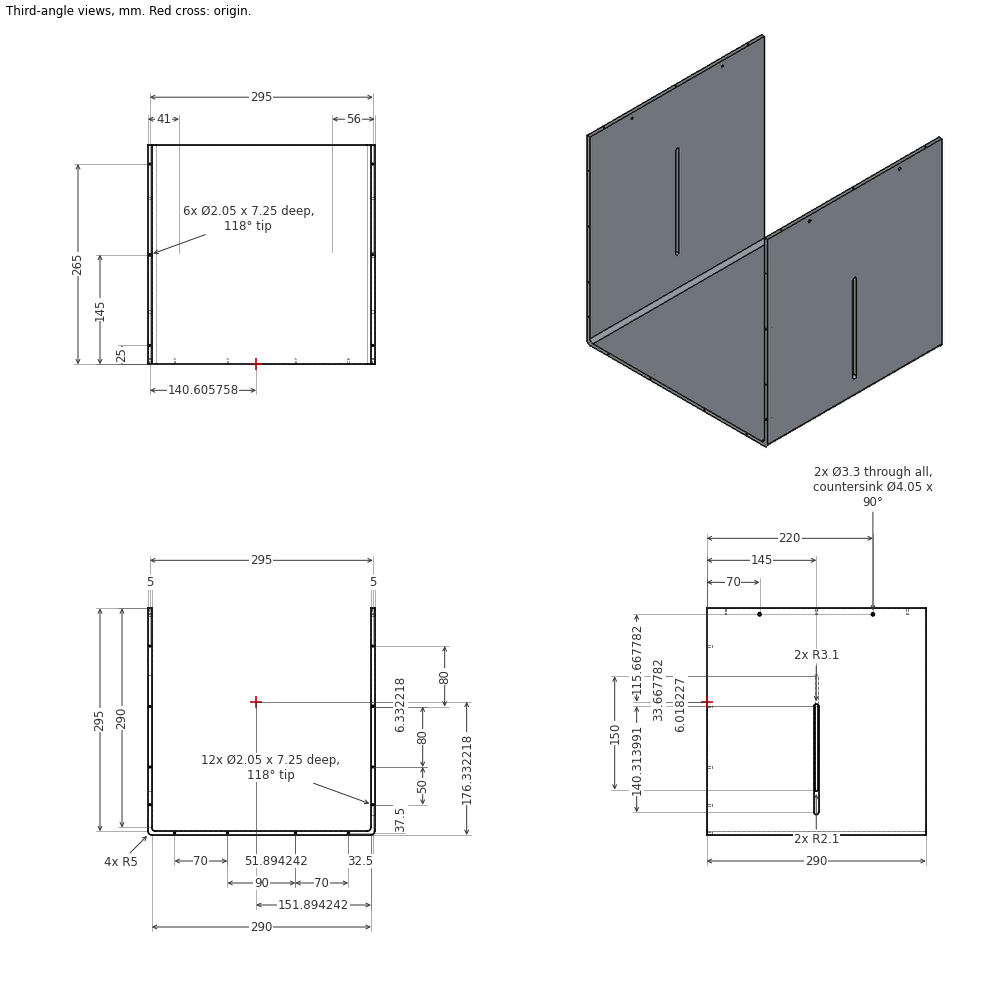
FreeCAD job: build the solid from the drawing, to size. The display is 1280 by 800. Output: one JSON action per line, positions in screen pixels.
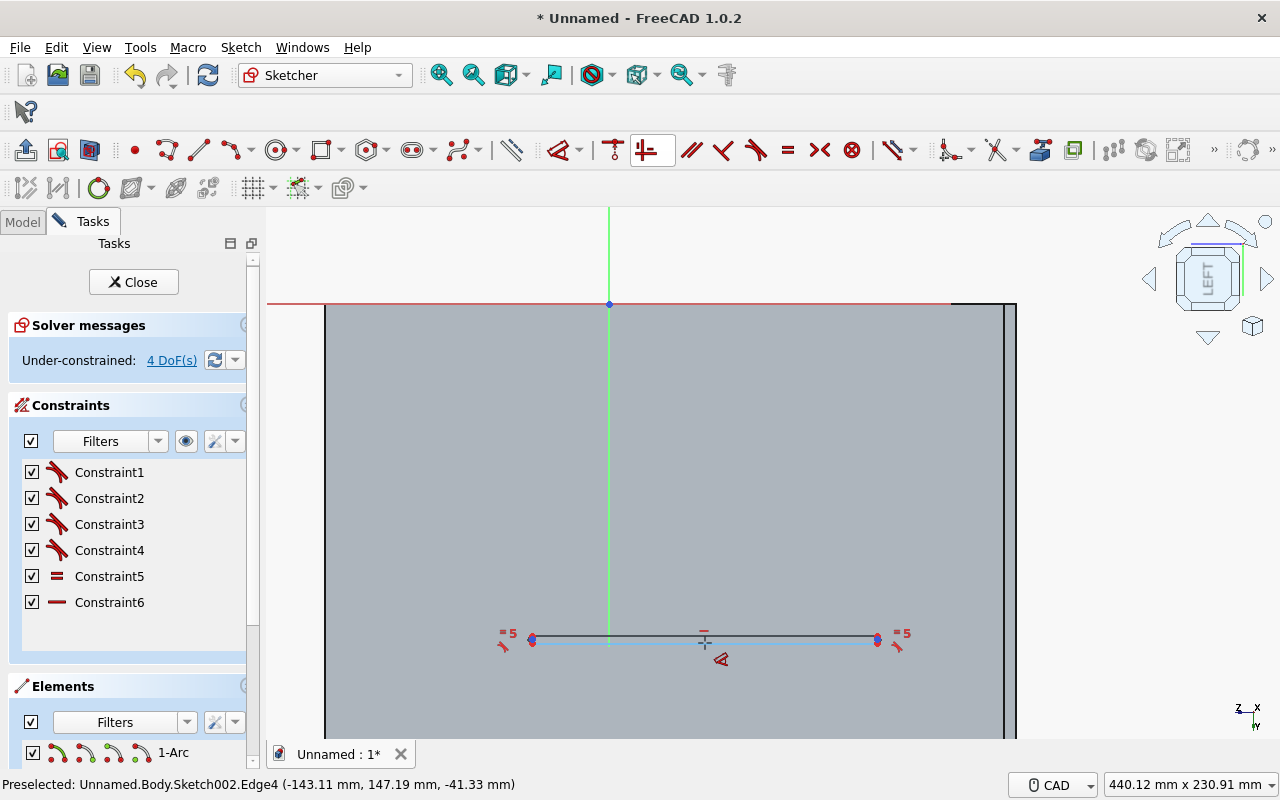
{"action": "scroll", "coordinate": [529, 638], "scroll_direction": "up", "scroll_amount": 11}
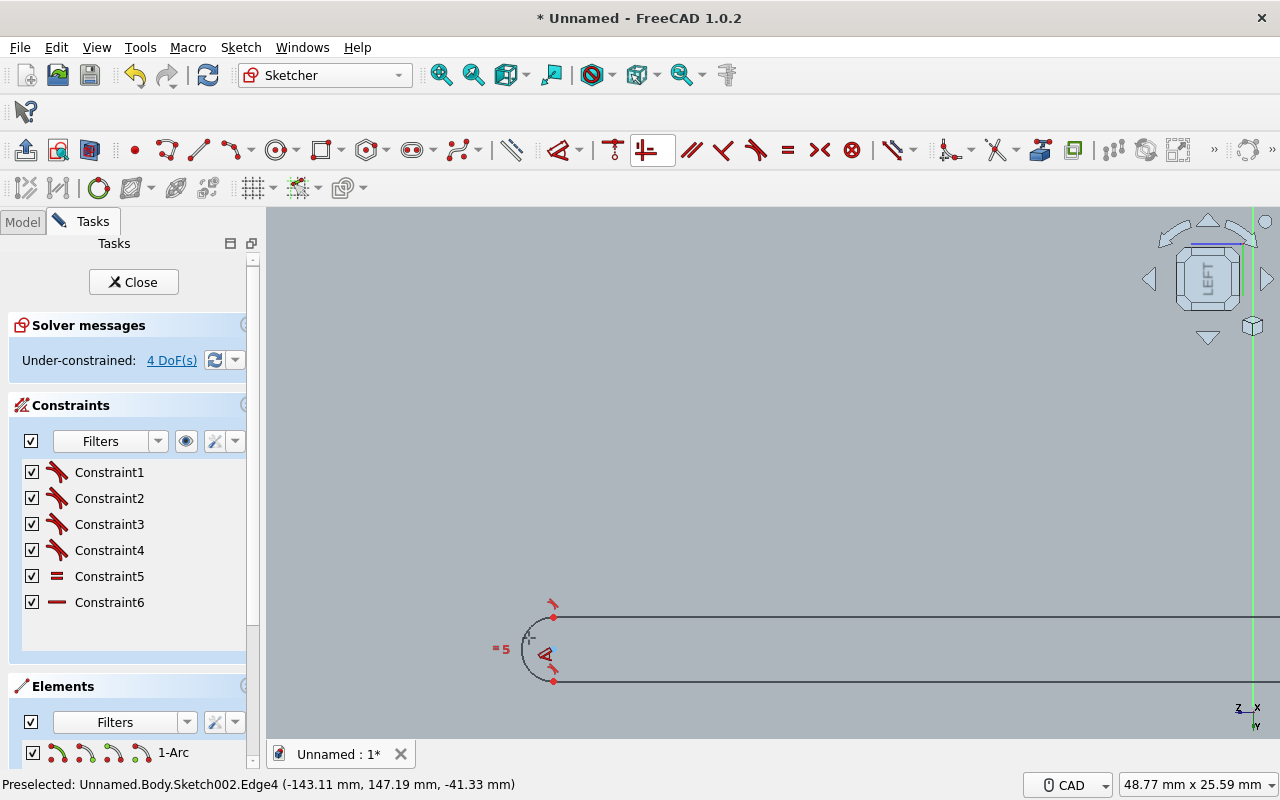
{"action": "left_click", "coordinate": [528, 631]}
{"action": "left_click", "coordinate": [502, 612]}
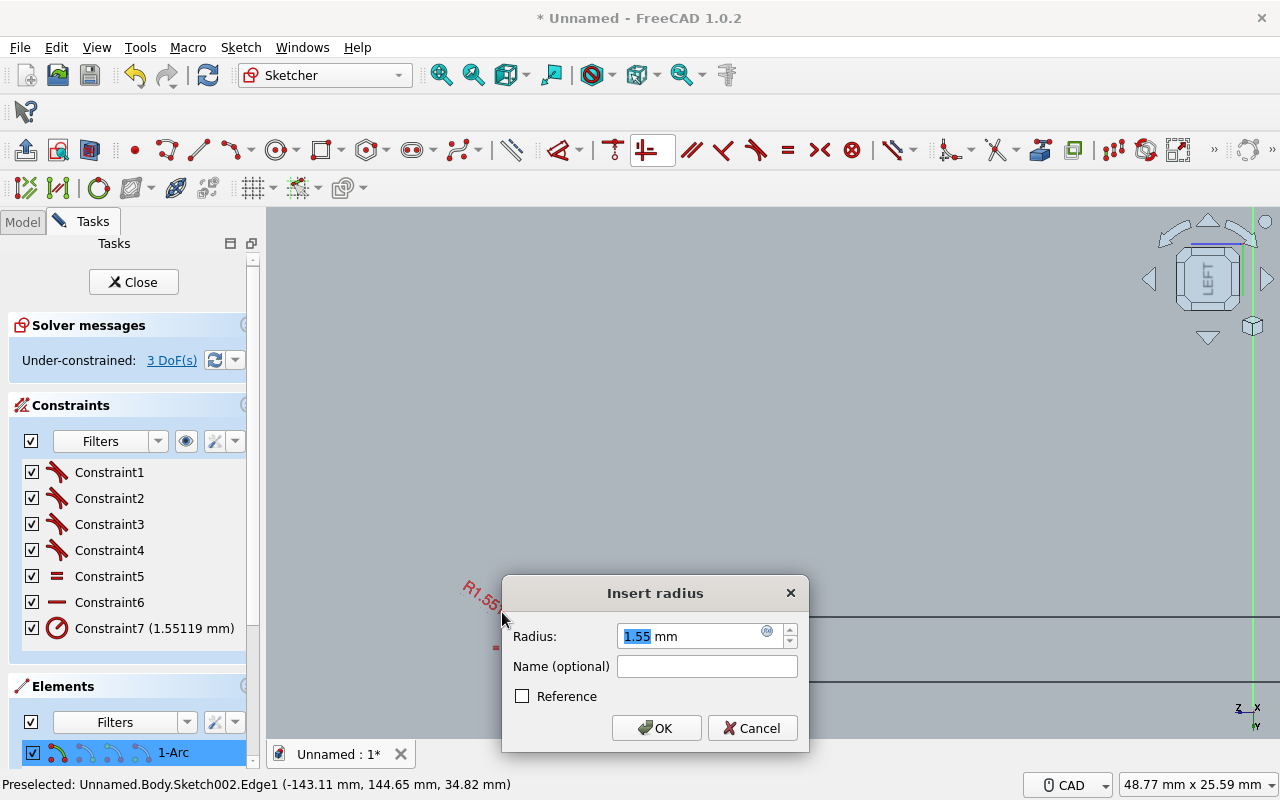
{"action": "type", "text": "2.1"}
{"action": "key", "text": "Return"}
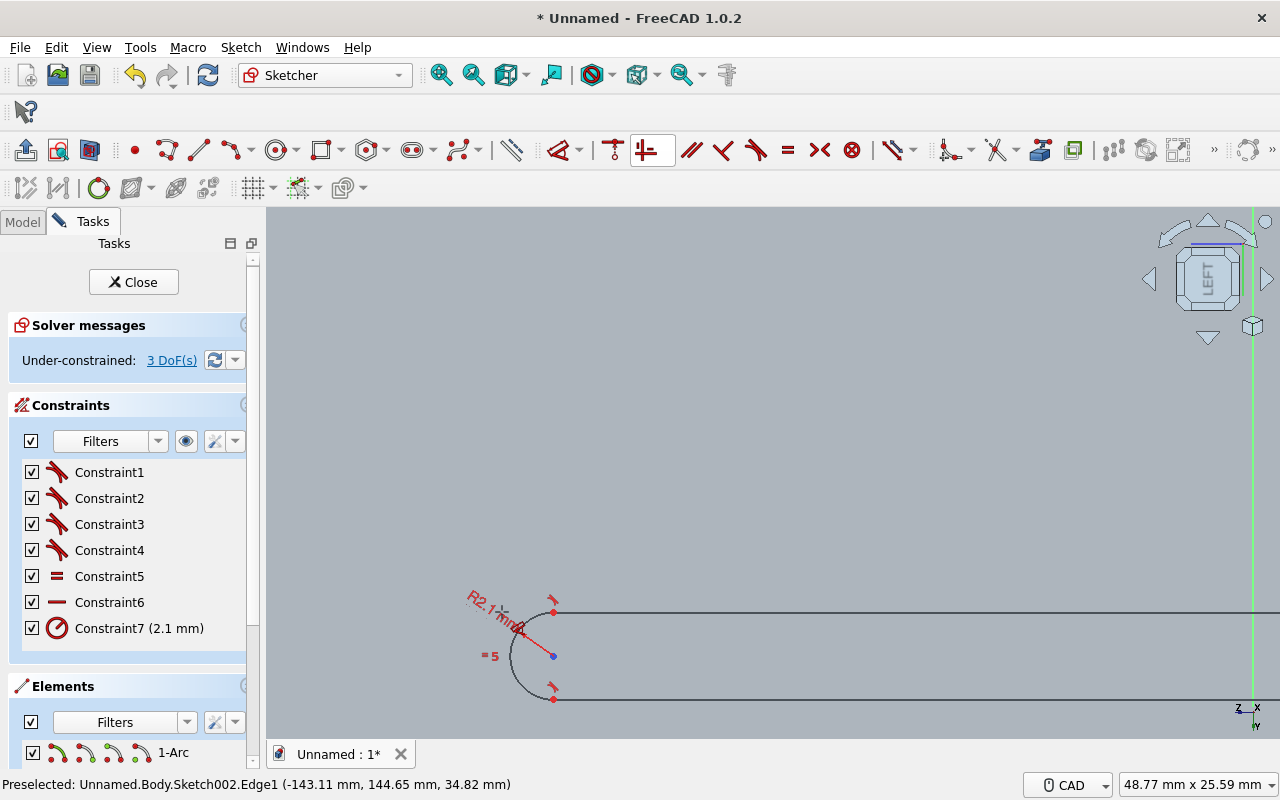
{"action": "scroll", "coordinate": [529, 638], "scroll_direction": "down", "scroll_amount": 11}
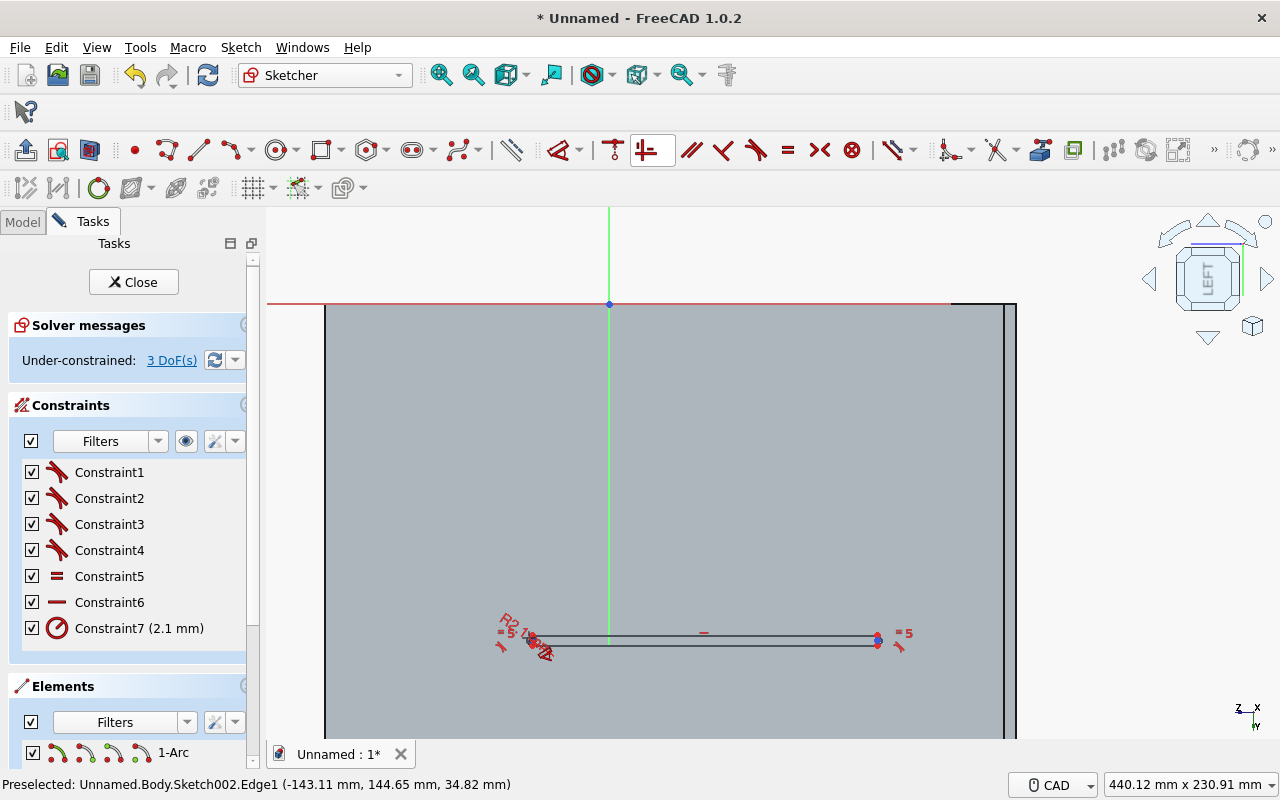
{"action": "scroll", "coordinate": [635, 636], "scroll_direction": "up", "scroll_amount": 2}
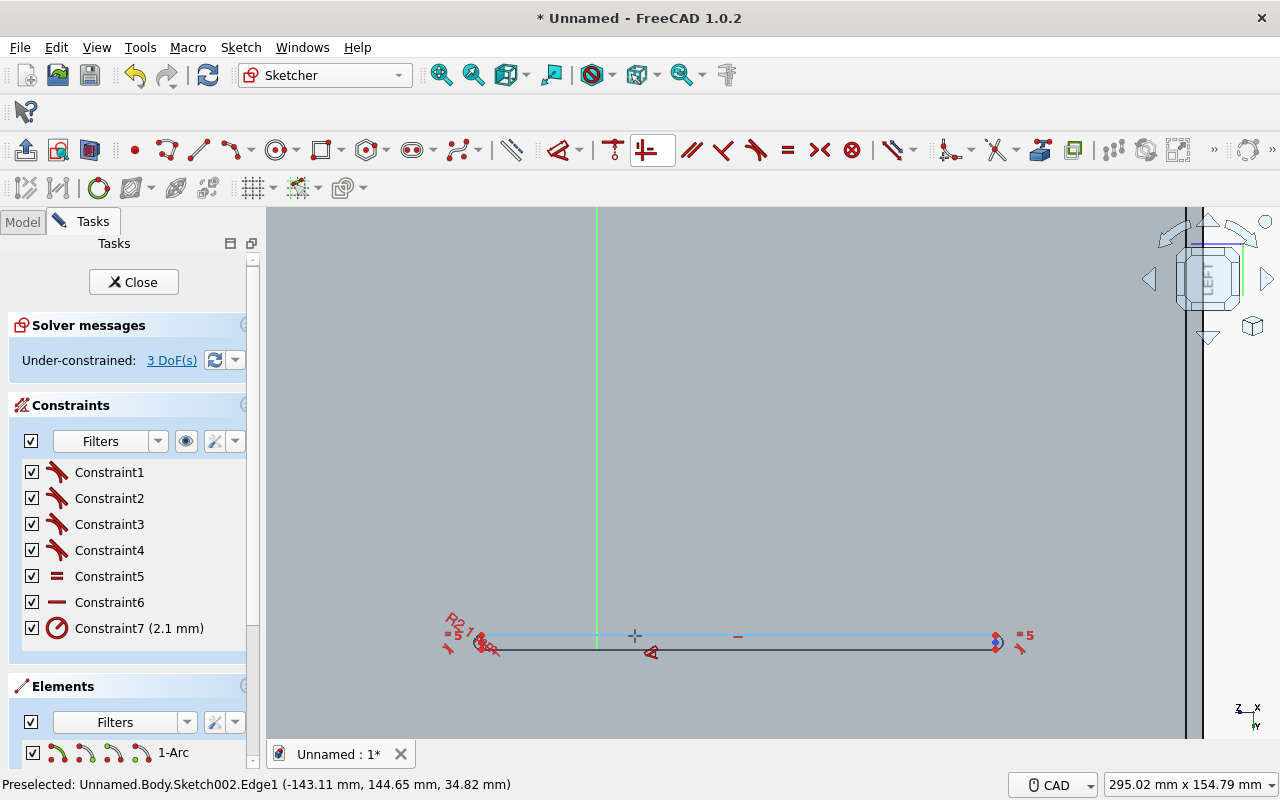
{"action": "left_click", "coordinate": [636, 635]}
{"action": "left_click", "coordinate": [739, 669]}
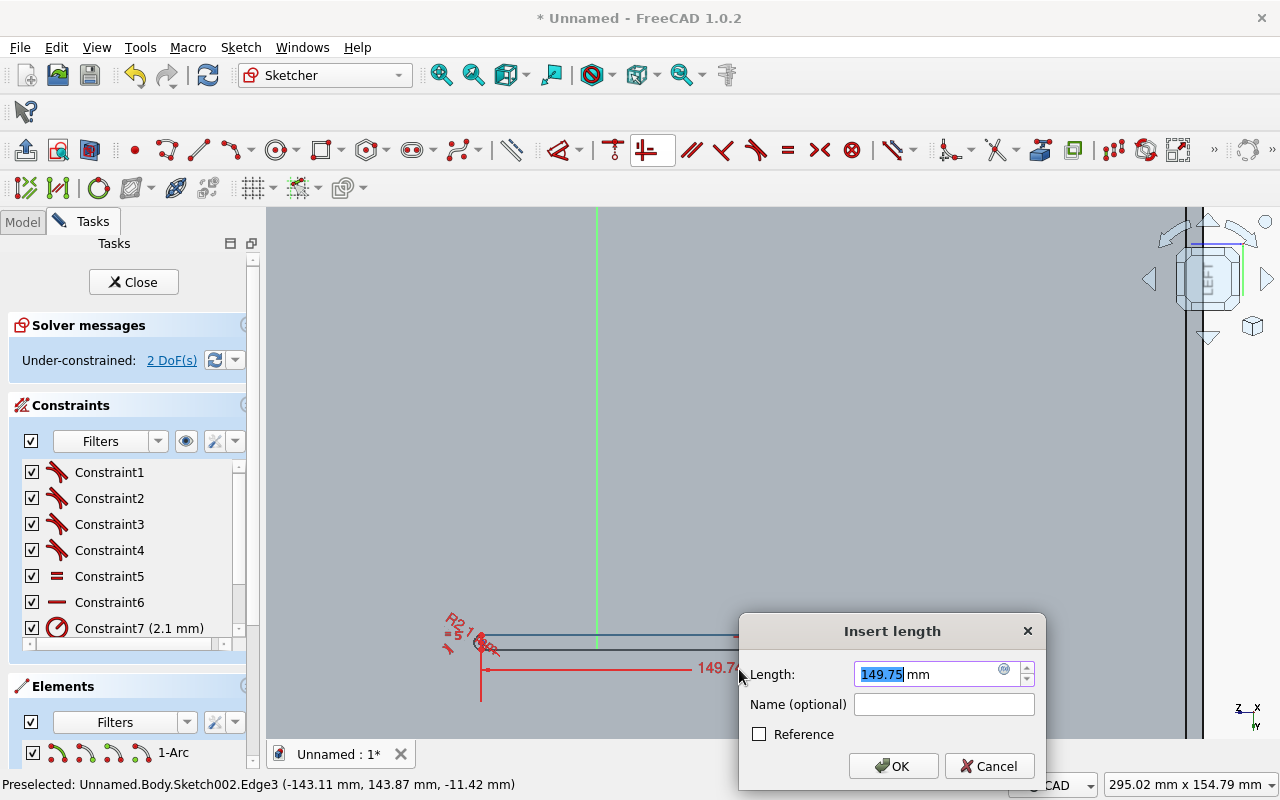
{"action": "type", "text": "150"}
{"action": "key", "text": "Return"}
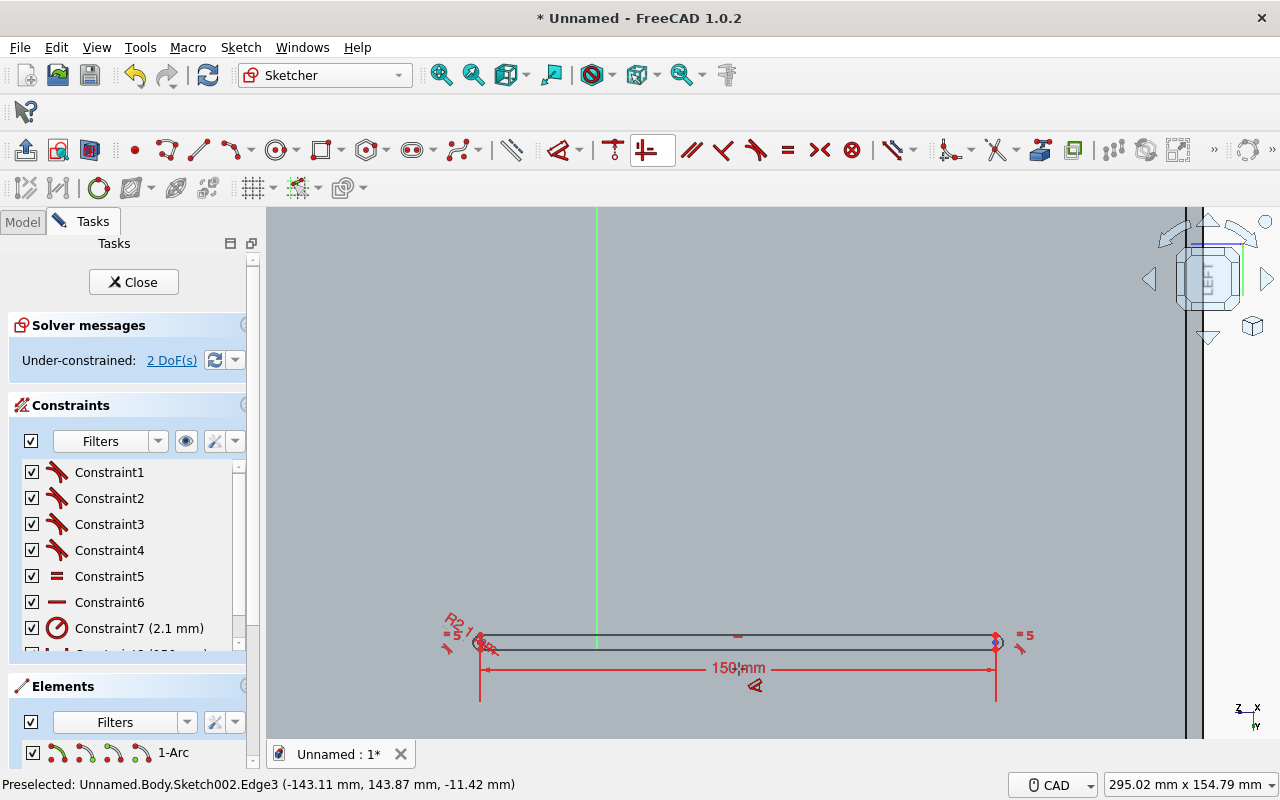
{"action": "scroll", "coordinate": [480, 643], "scroll_direction": "up", "scroll_amount": 3}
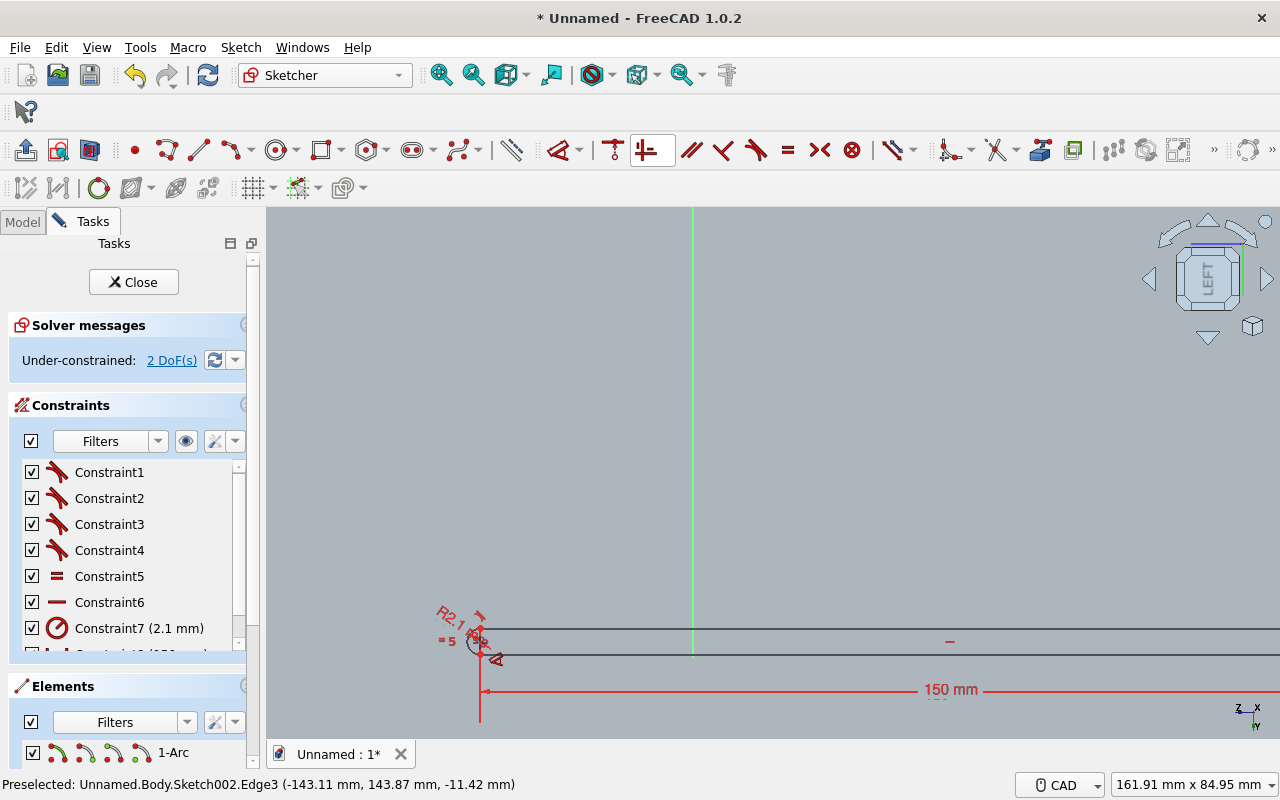
{"action": "left_click", "coordinate": [480, 642]}
{"action": "left_click", "coordinate": [446, 438]}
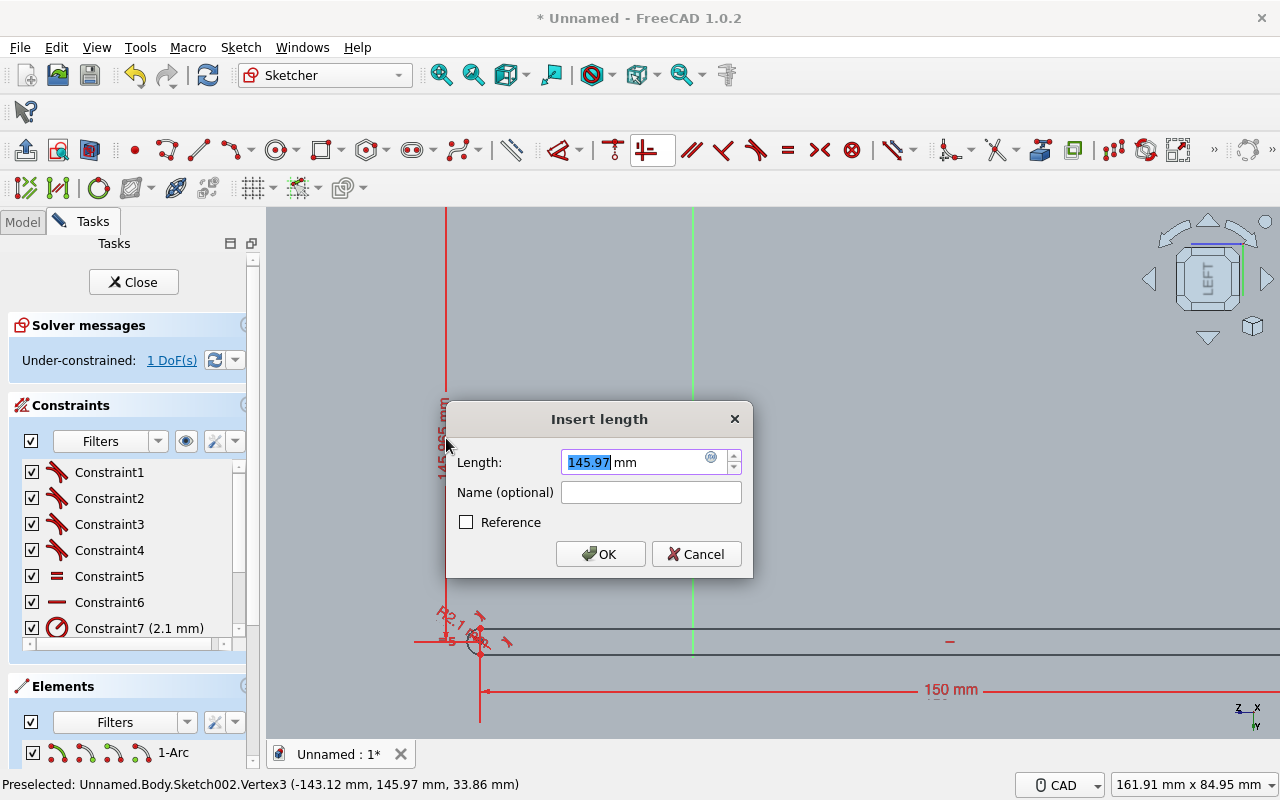
{"action": "type", "text": "145"}
{"action": "key", "text": "Return"}